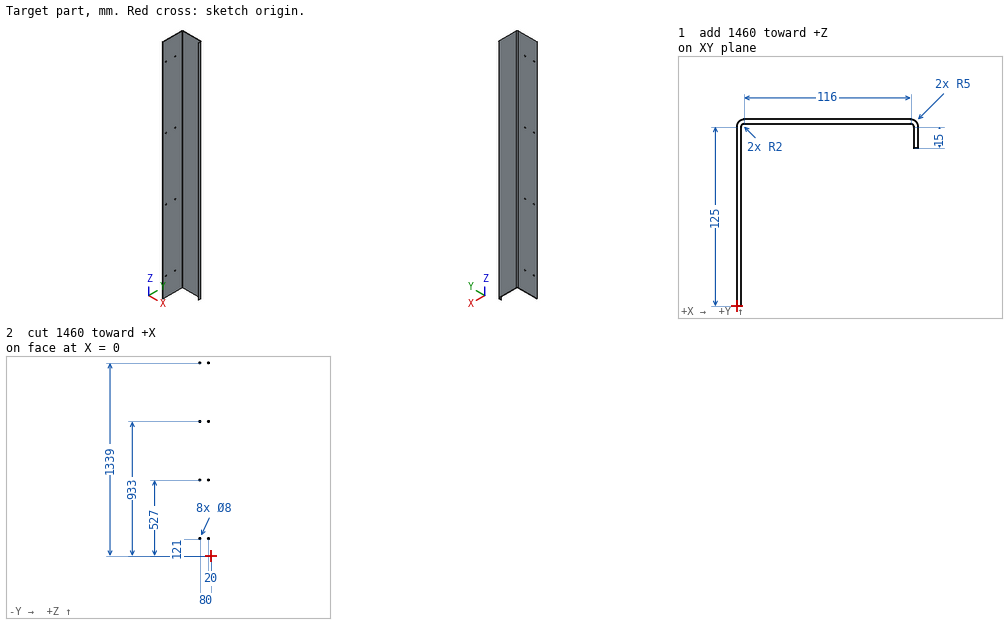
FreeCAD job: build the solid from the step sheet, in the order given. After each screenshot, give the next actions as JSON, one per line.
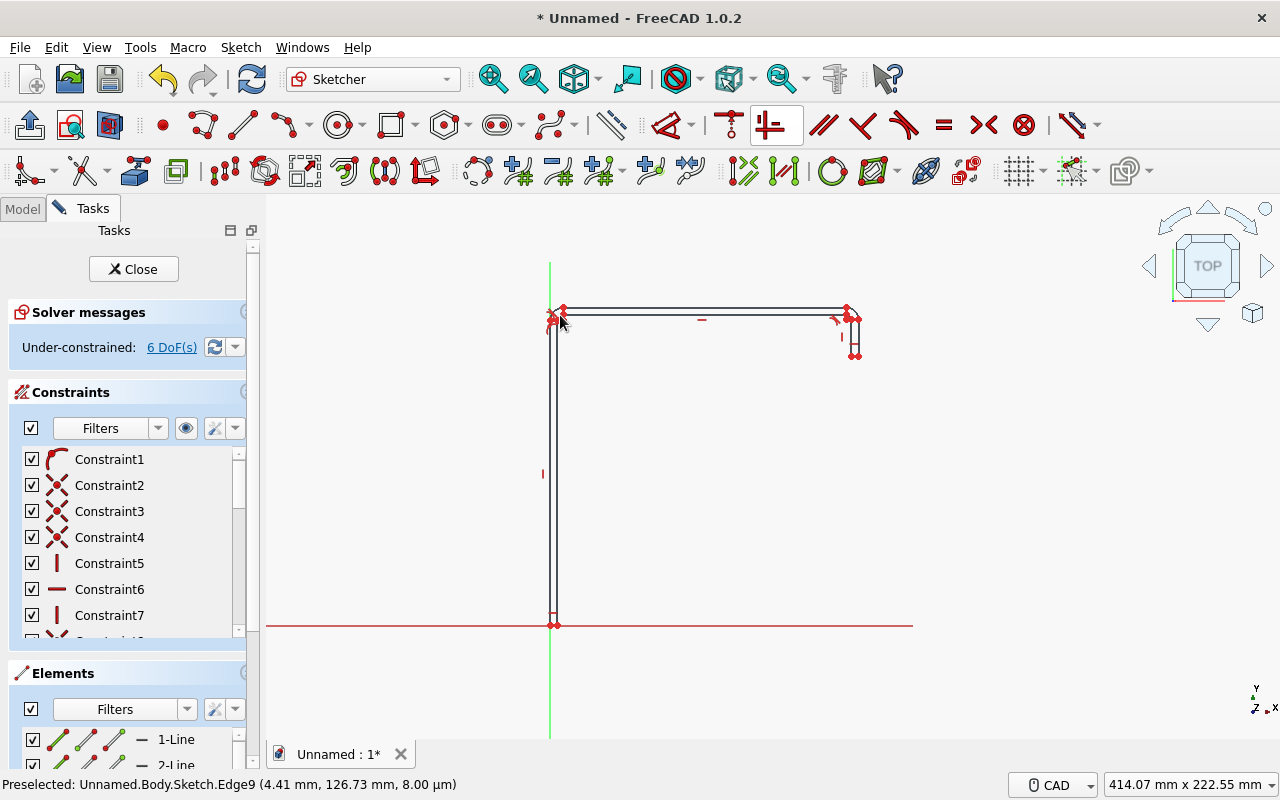
{"action": "scroll", "coordinate": [851, 318], "scroll_direction": "up", "scroll_amount": 9}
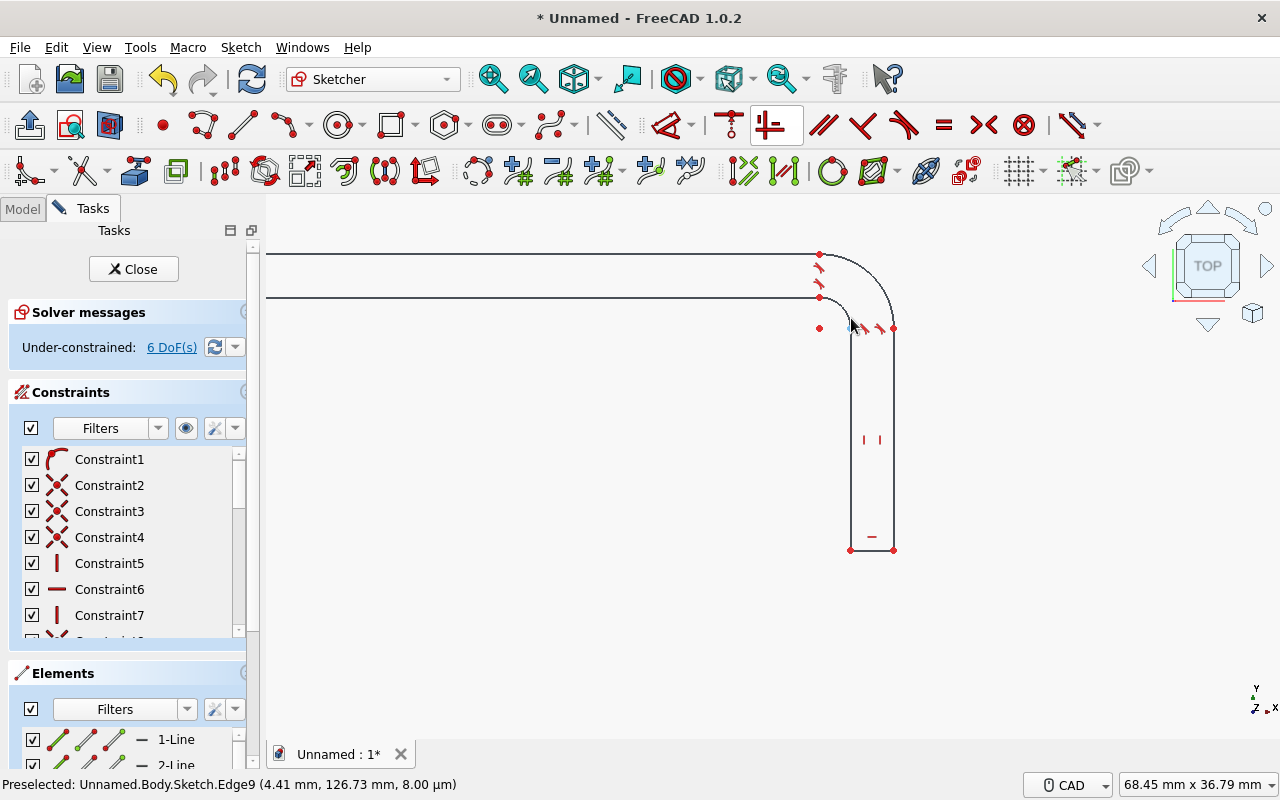
{"action": "left_click", "coordinate": [847, 314]}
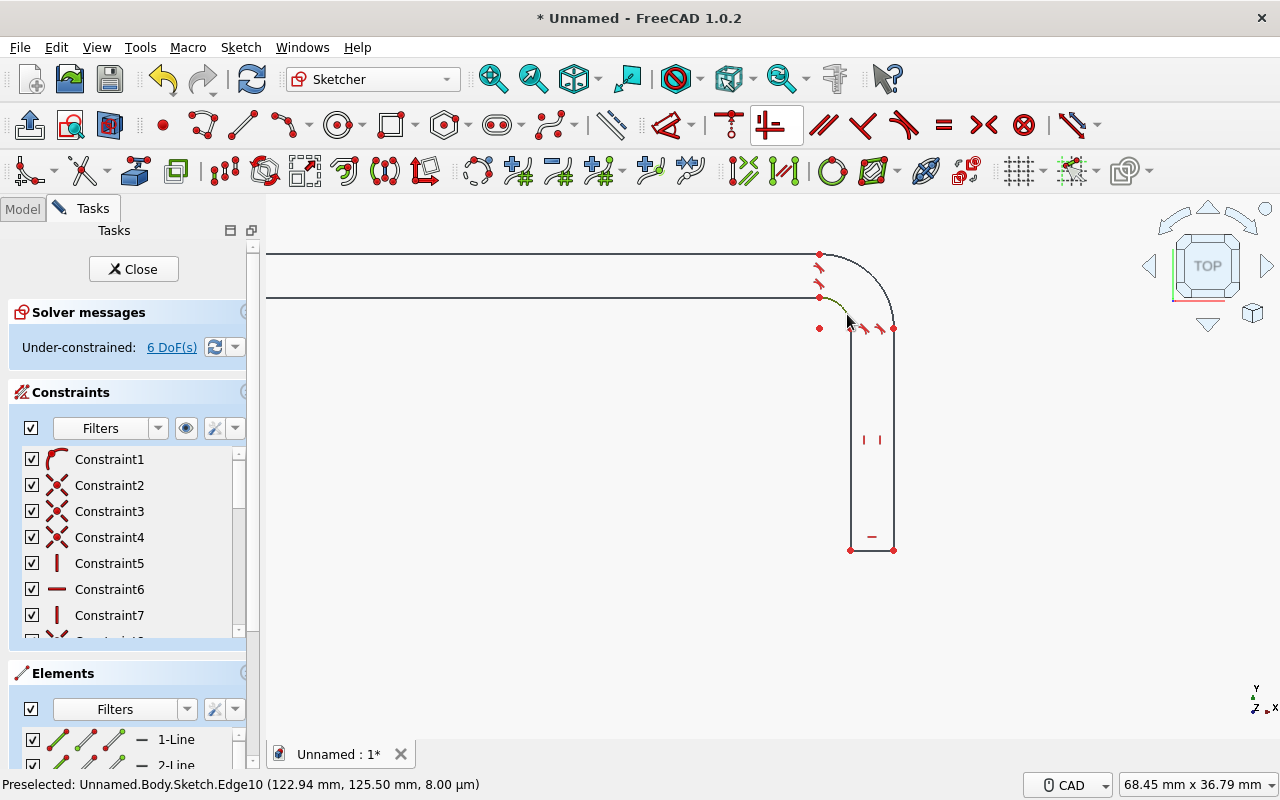
{"action": "key", "text": "e"}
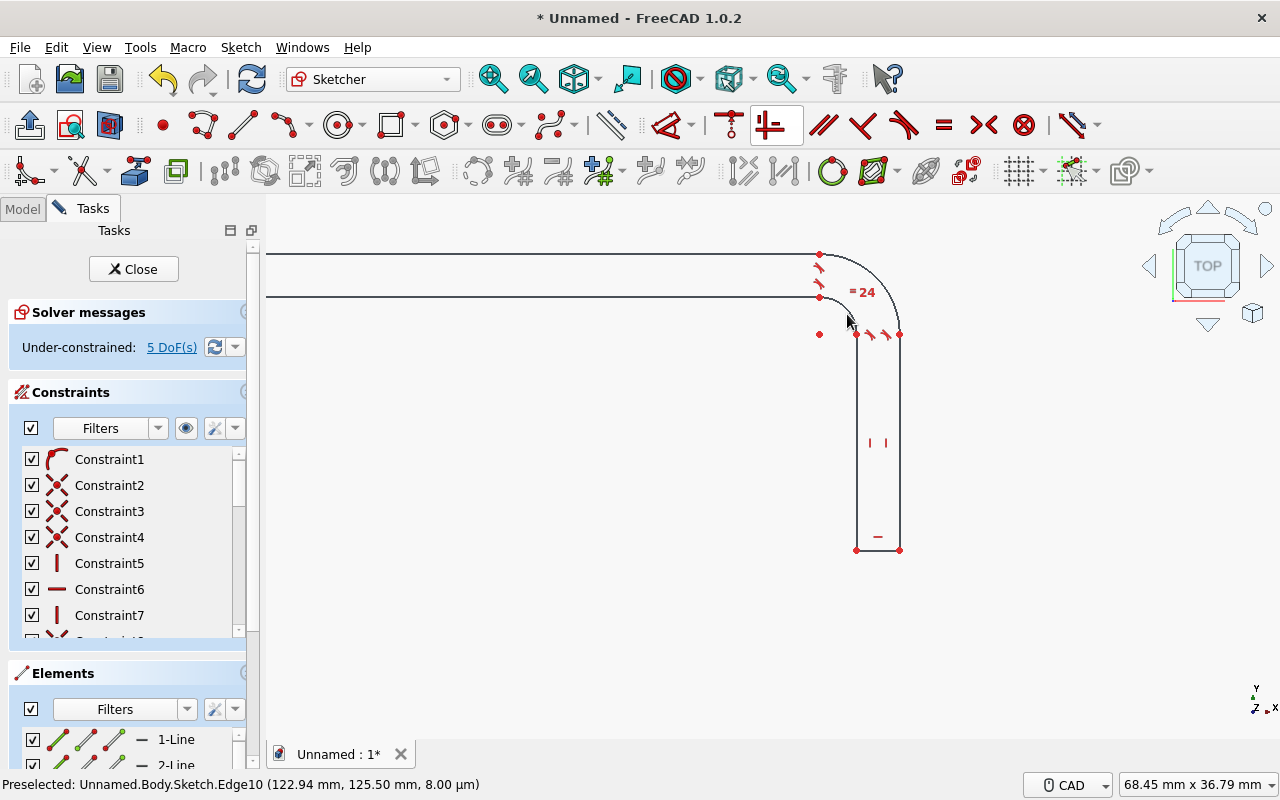
{"action": "scroll", "coordinate": [852, 318], "scroll_direction": "down", "scroll_amount": 9}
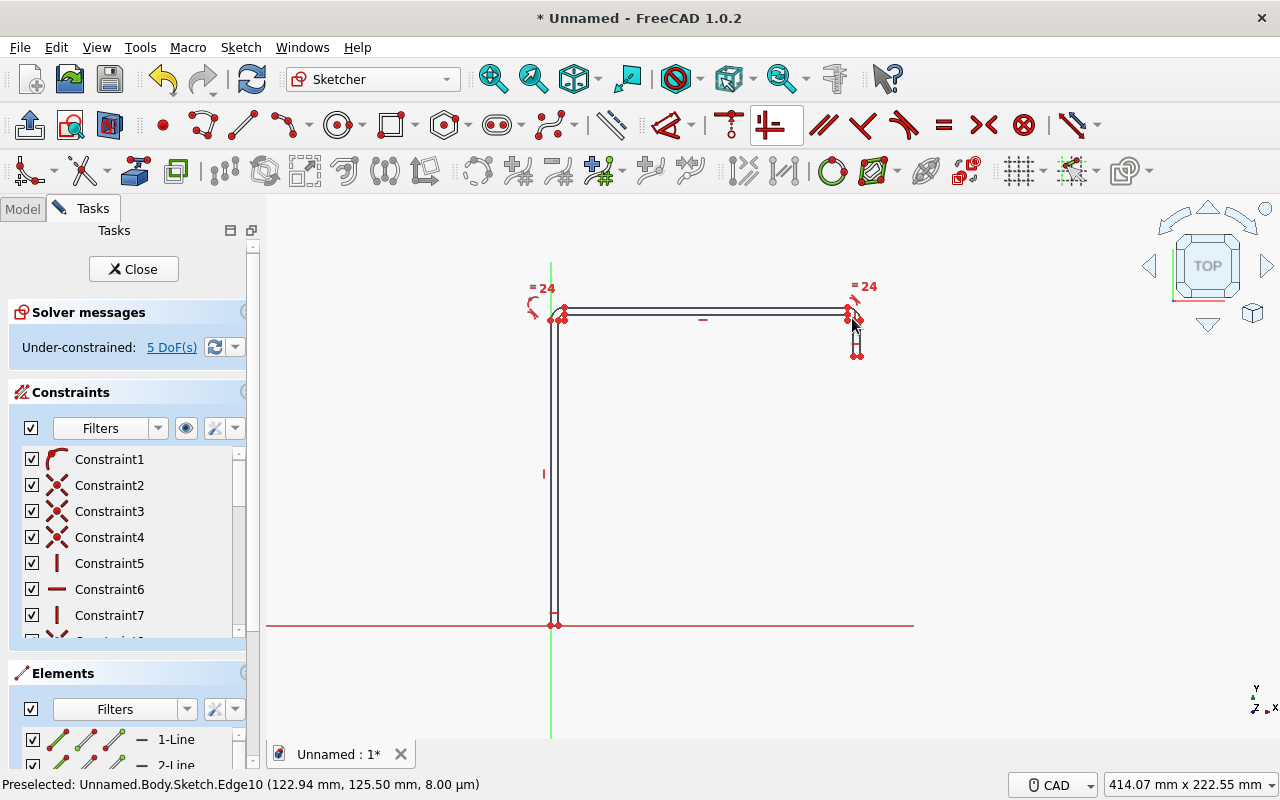
{"action": "scroll", "coordinate": [561, 315], "scroll_direction": "up", "scroll_amount": 11}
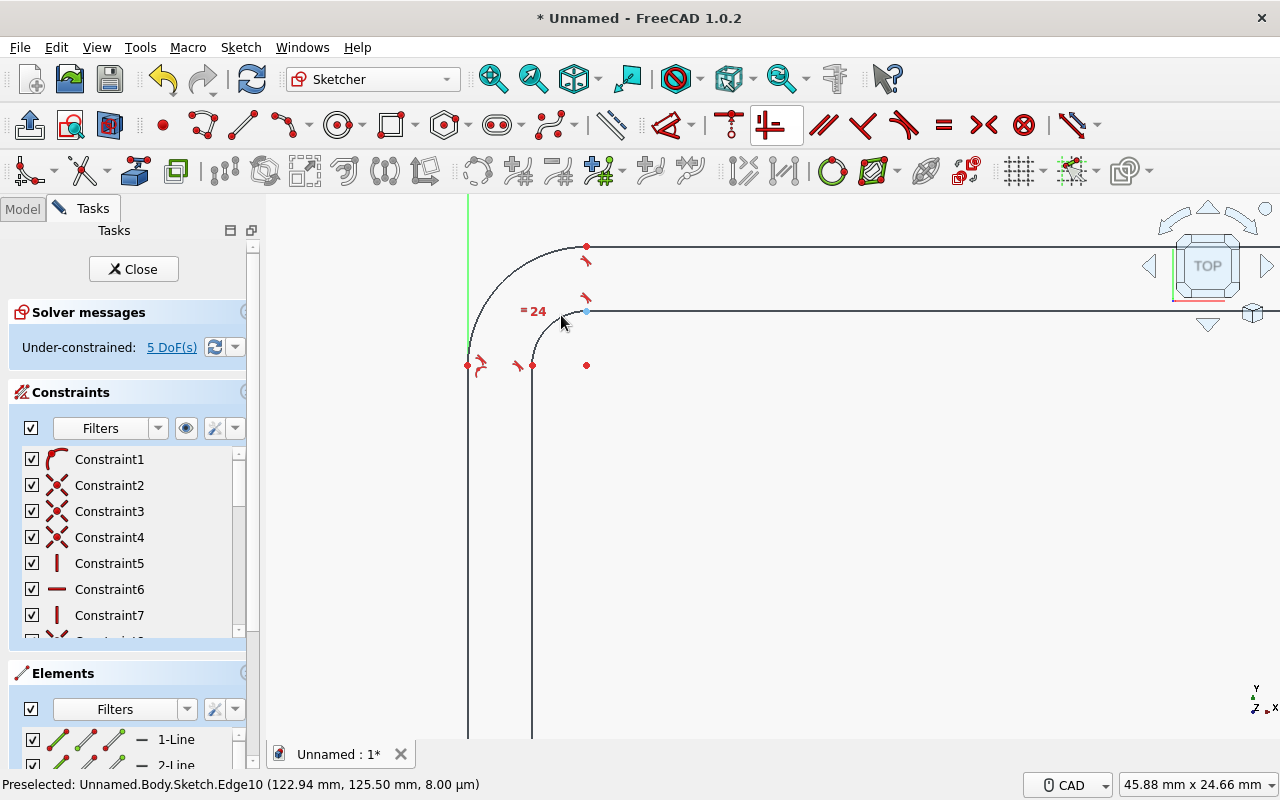
{"action": "left_click", "coordinate": [562, 317]}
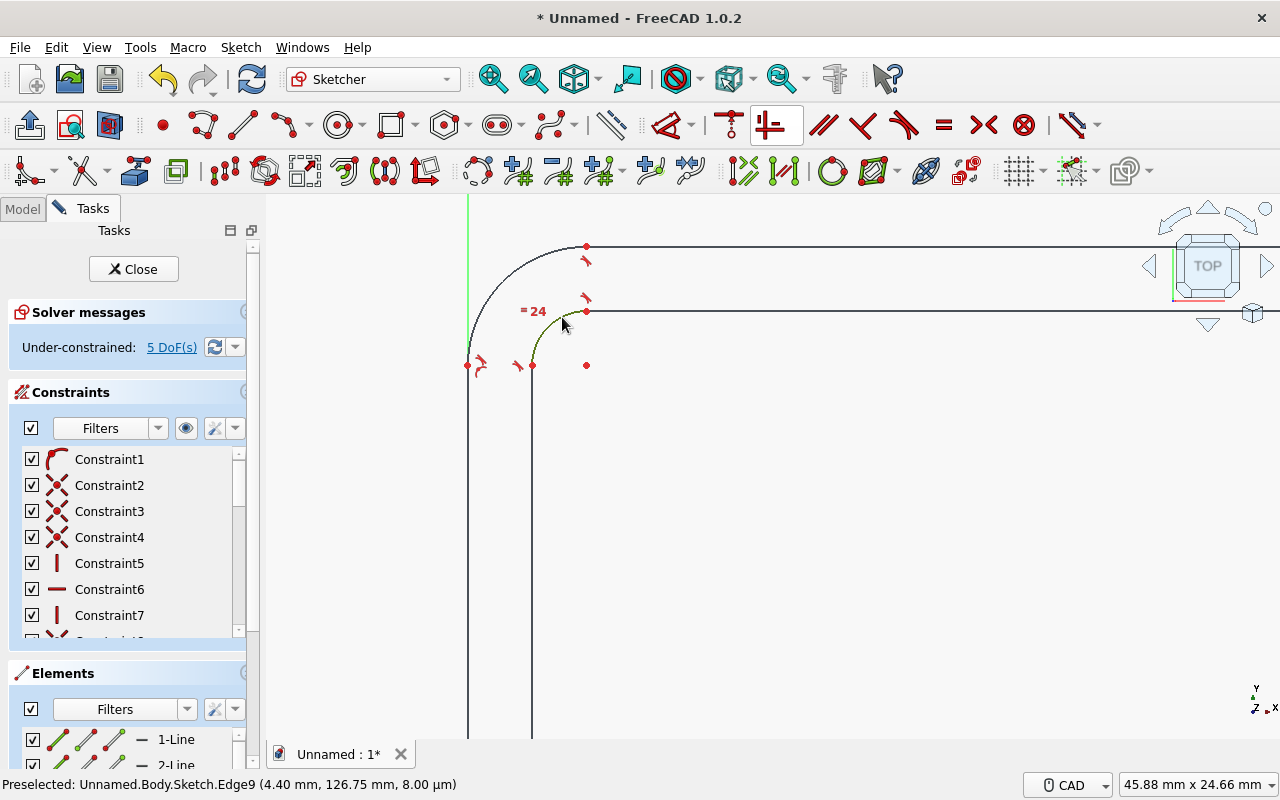
{"action": "left_click", "coordinate": [694, 126]}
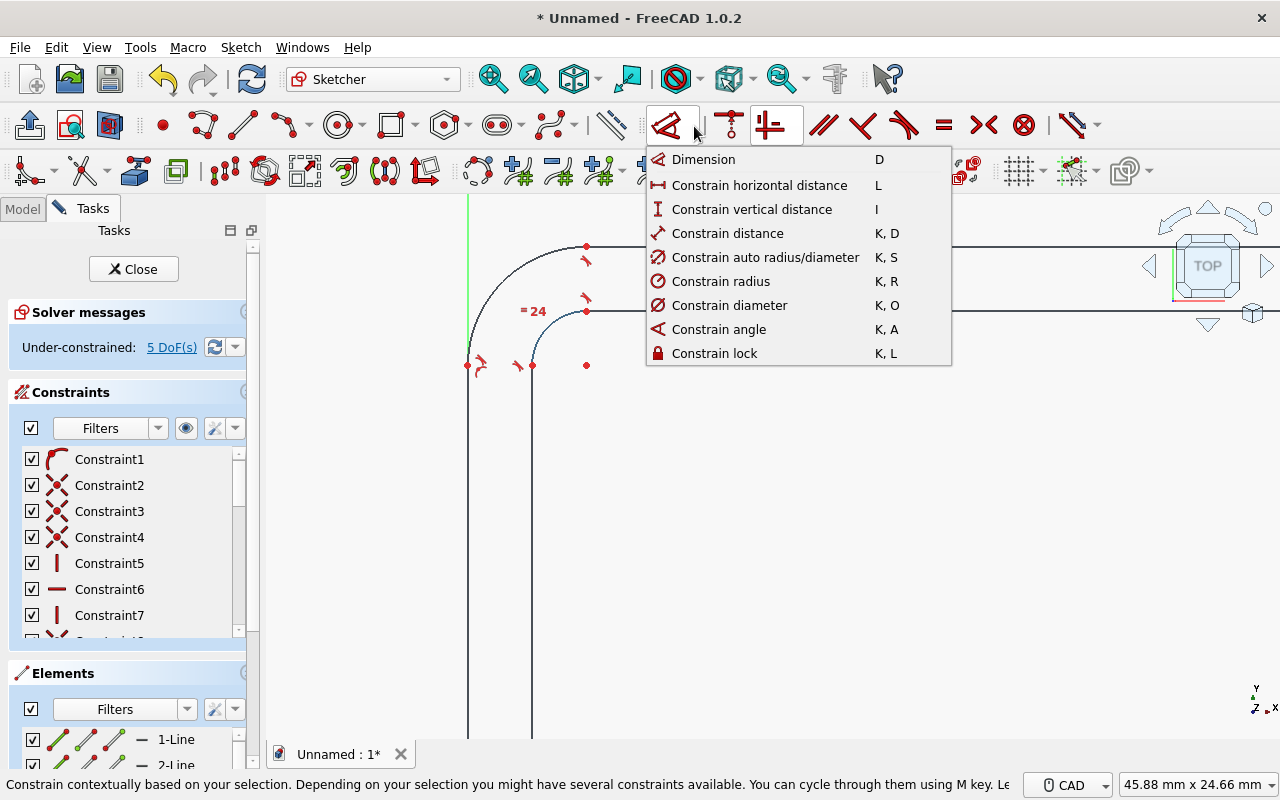
{"action": "left_click", "coordinate": [799, 281]}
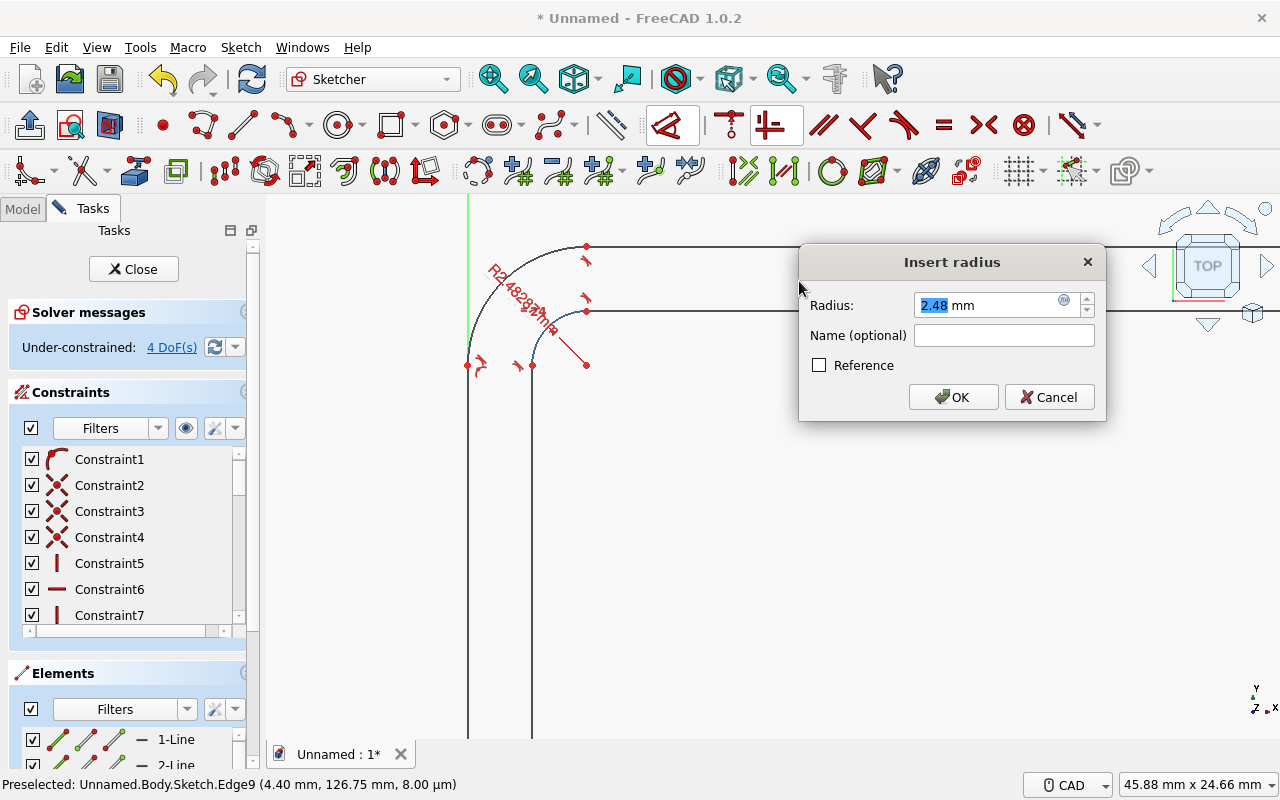
{"action": "type", "text": "2"}
{"action": "key", "text": "Return"}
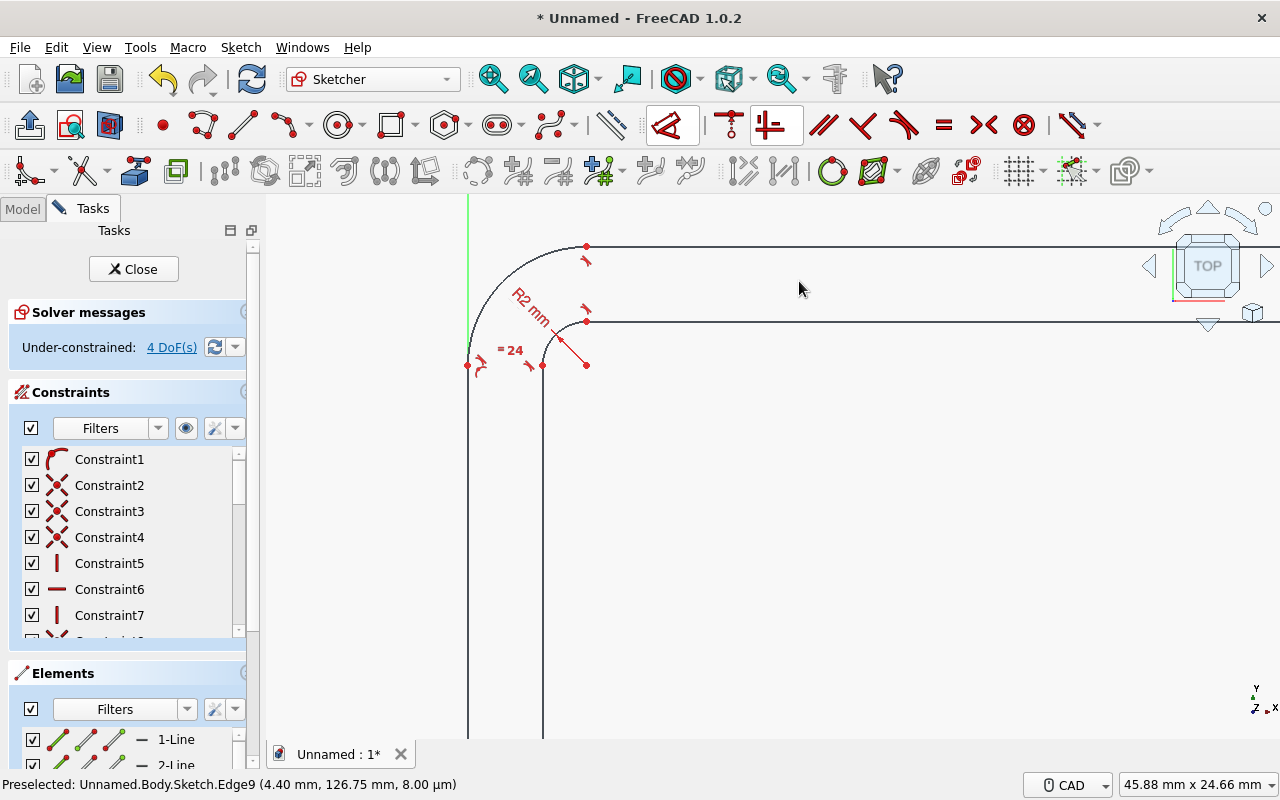
{"action": "scroll", "coordinate": [560, 315], "scroll_direction": "down", "scroll_amount": 11}